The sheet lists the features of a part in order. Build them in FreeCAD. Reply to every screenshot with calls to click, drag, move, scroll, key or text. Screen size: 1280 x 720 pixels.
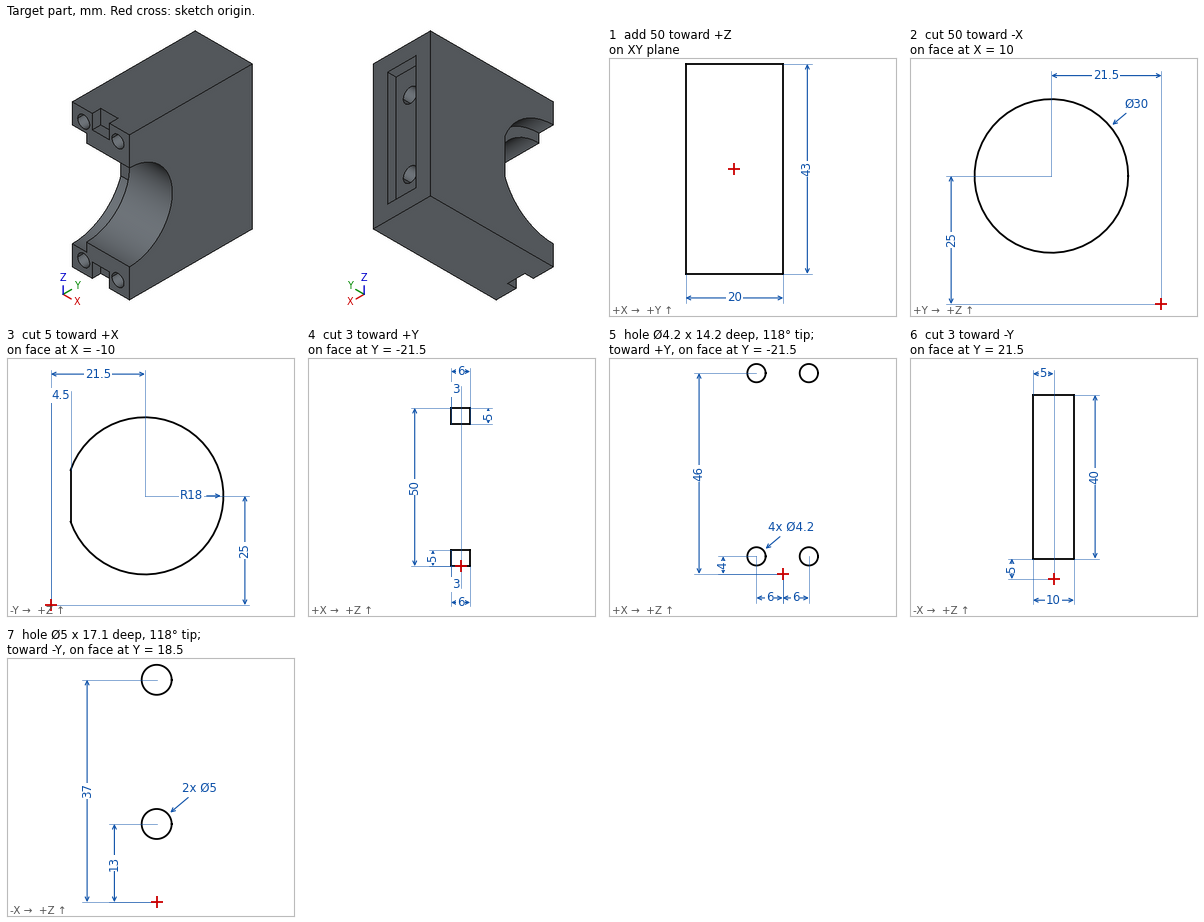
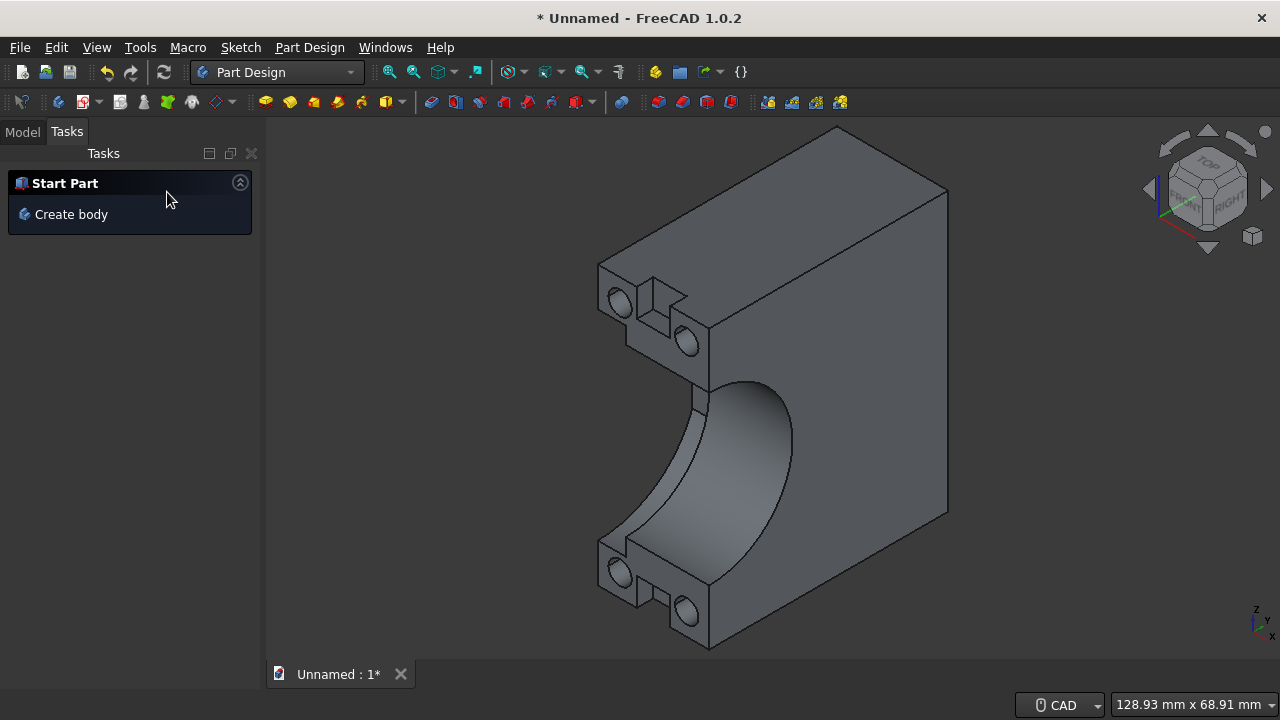
key(4)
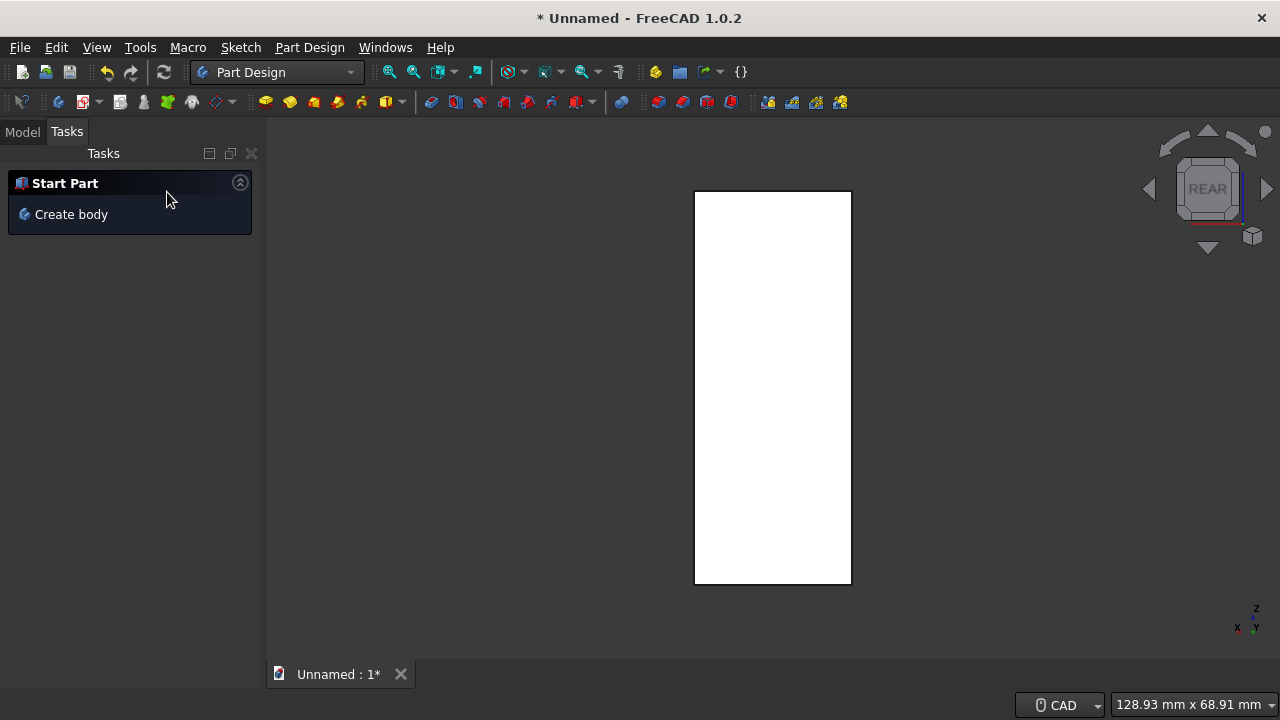
click(773, 275)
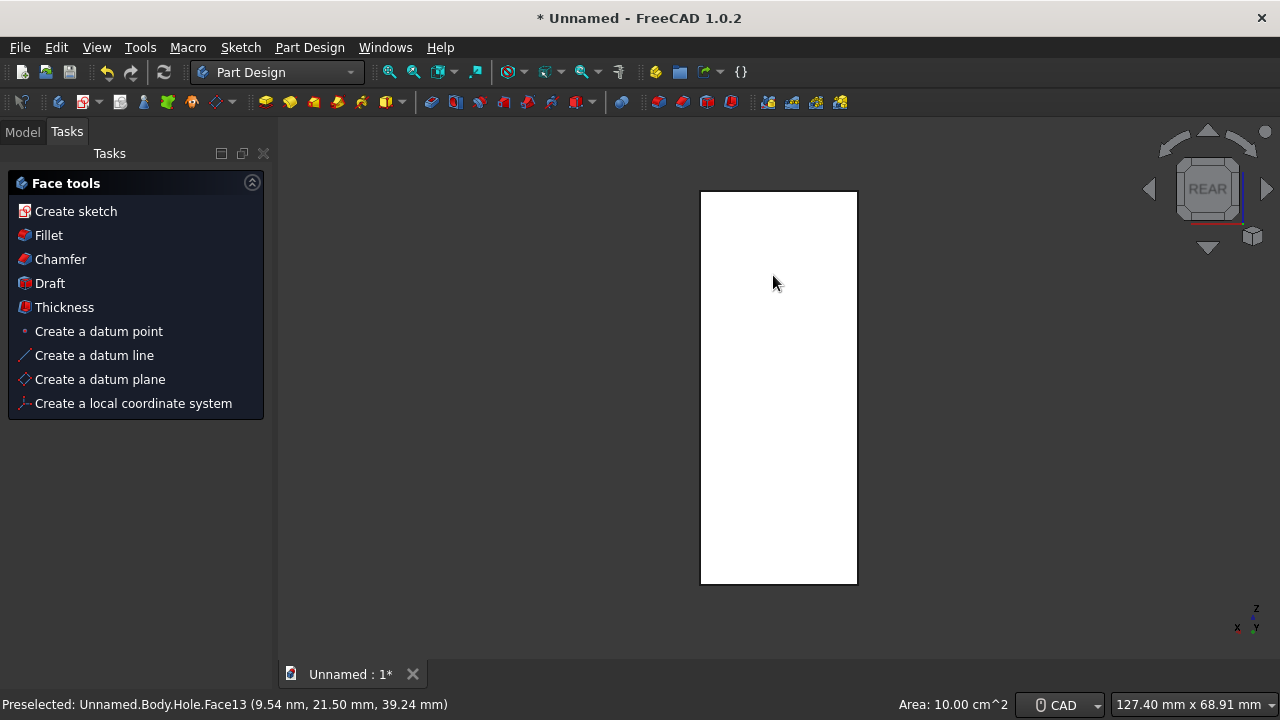
click(84, 102)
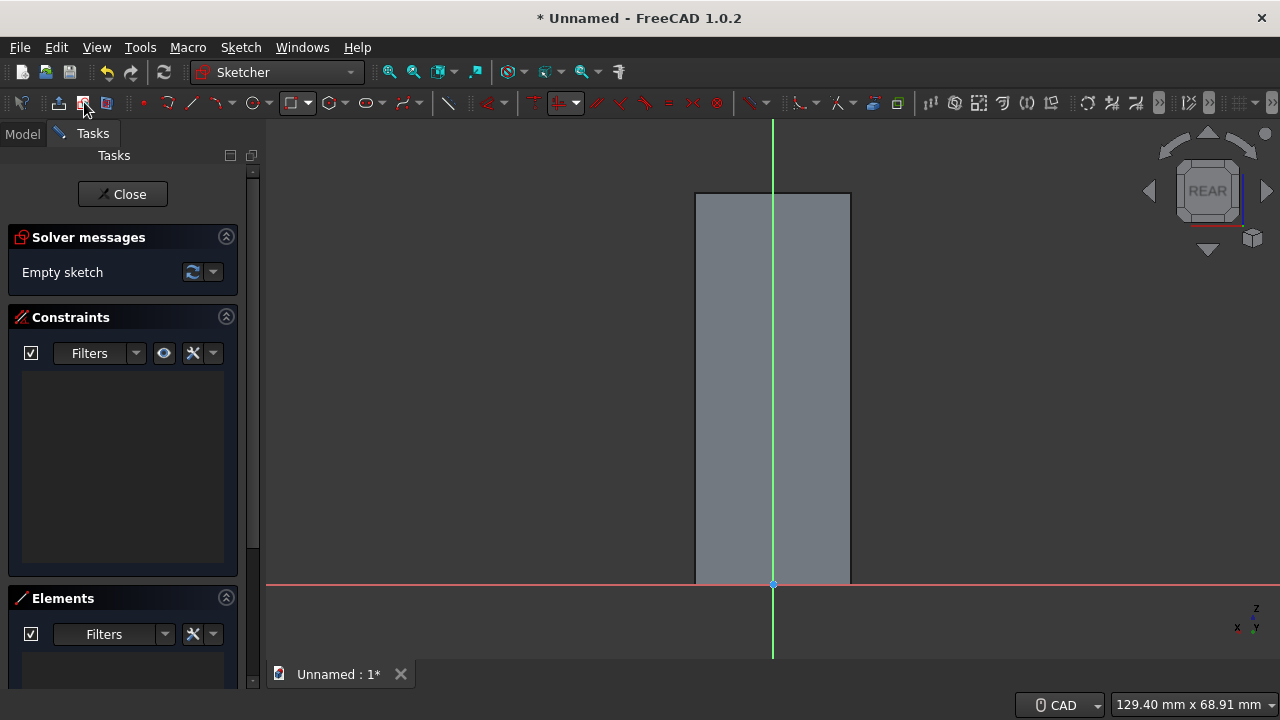
key(g)
key(r)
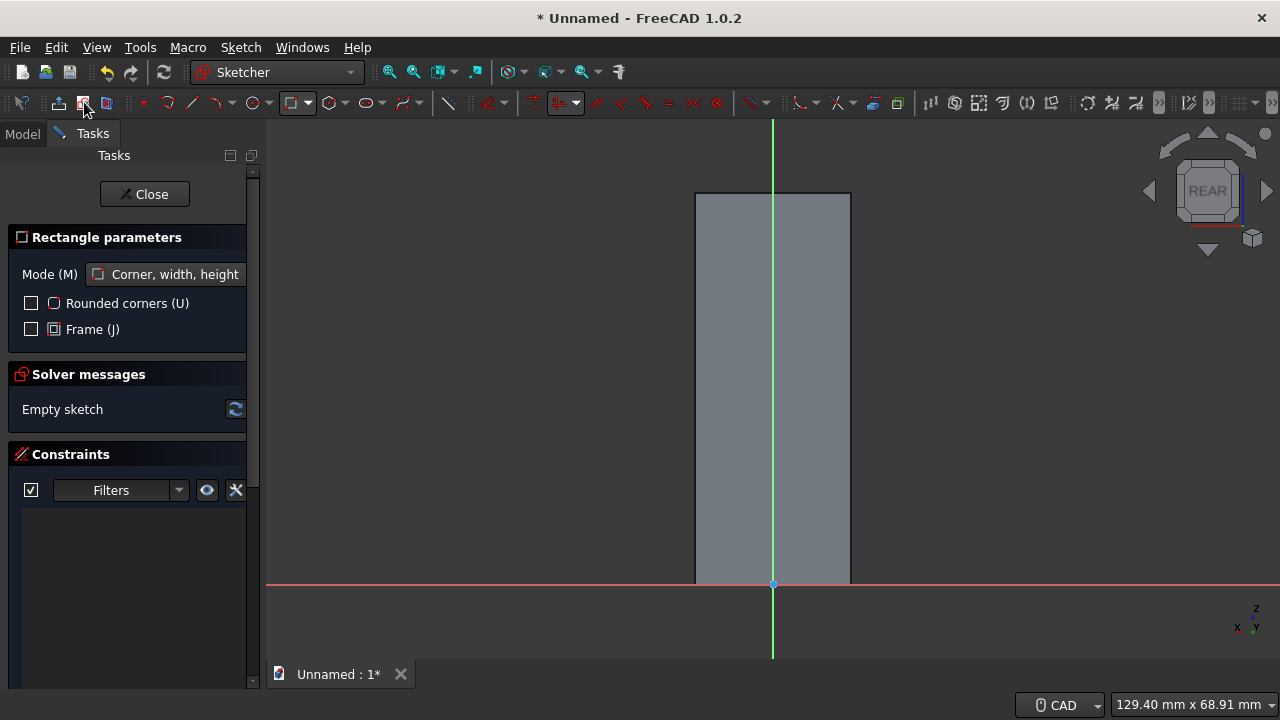
click(734, 232)
move(812, 546)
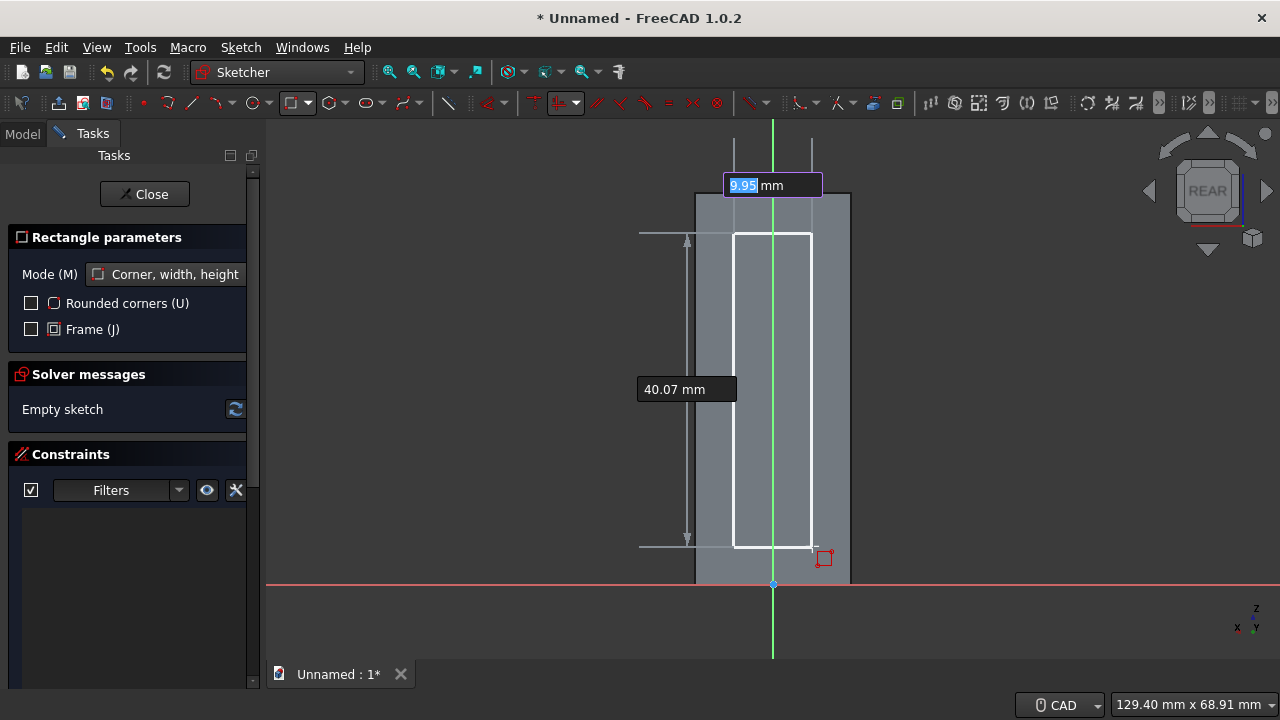
text(10)
key(Tab)
text(40)
key(Return)
key(Escape)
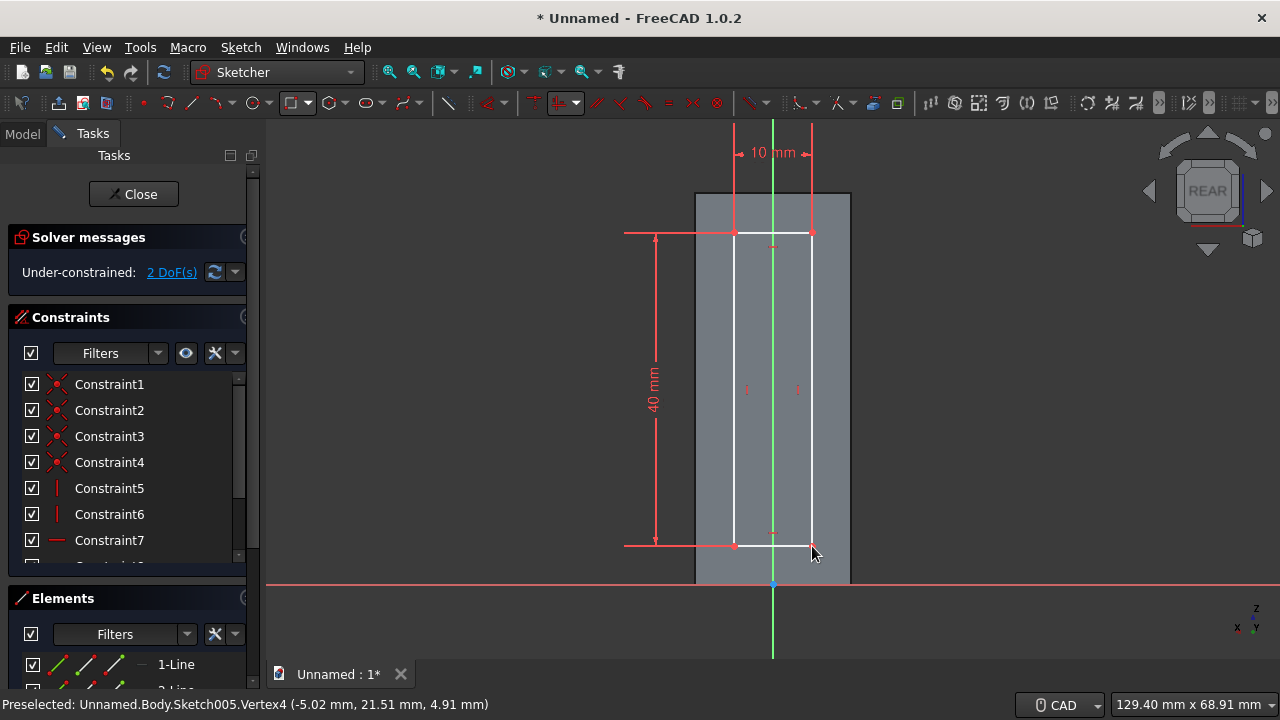
click(488, 104)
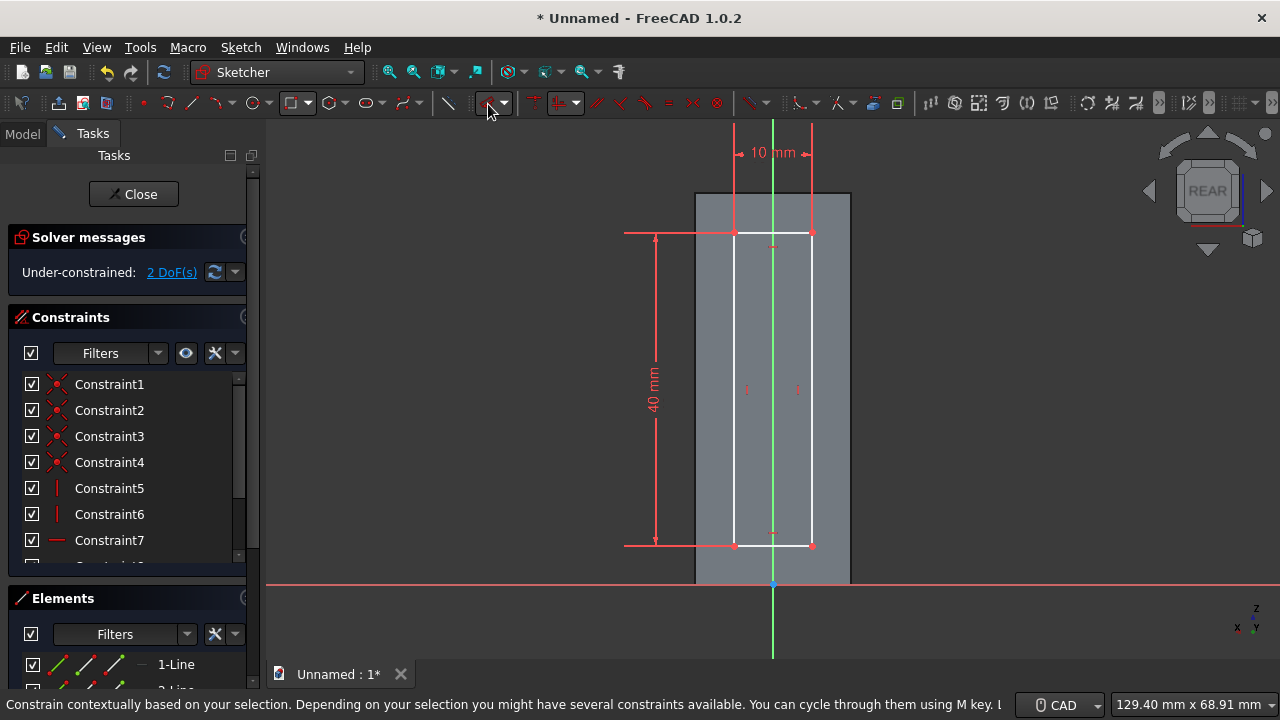
click(734, 233)
click(754, 619)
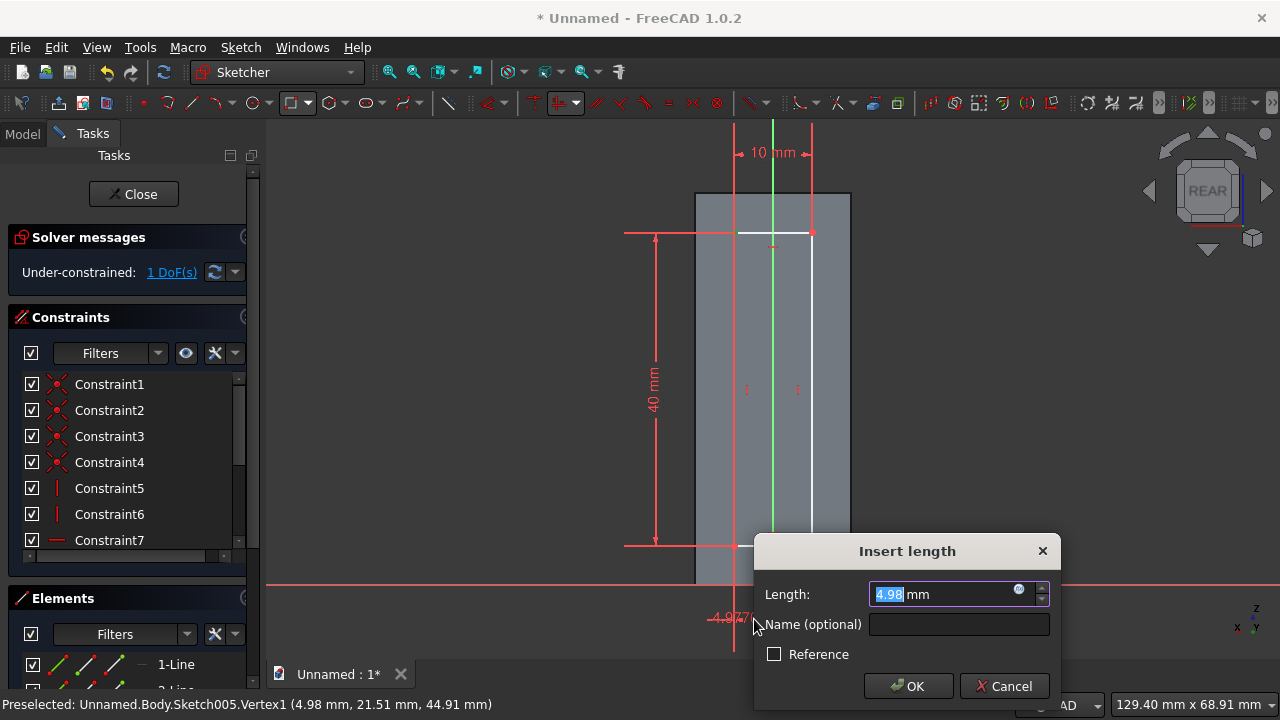
text(5)
key(Return)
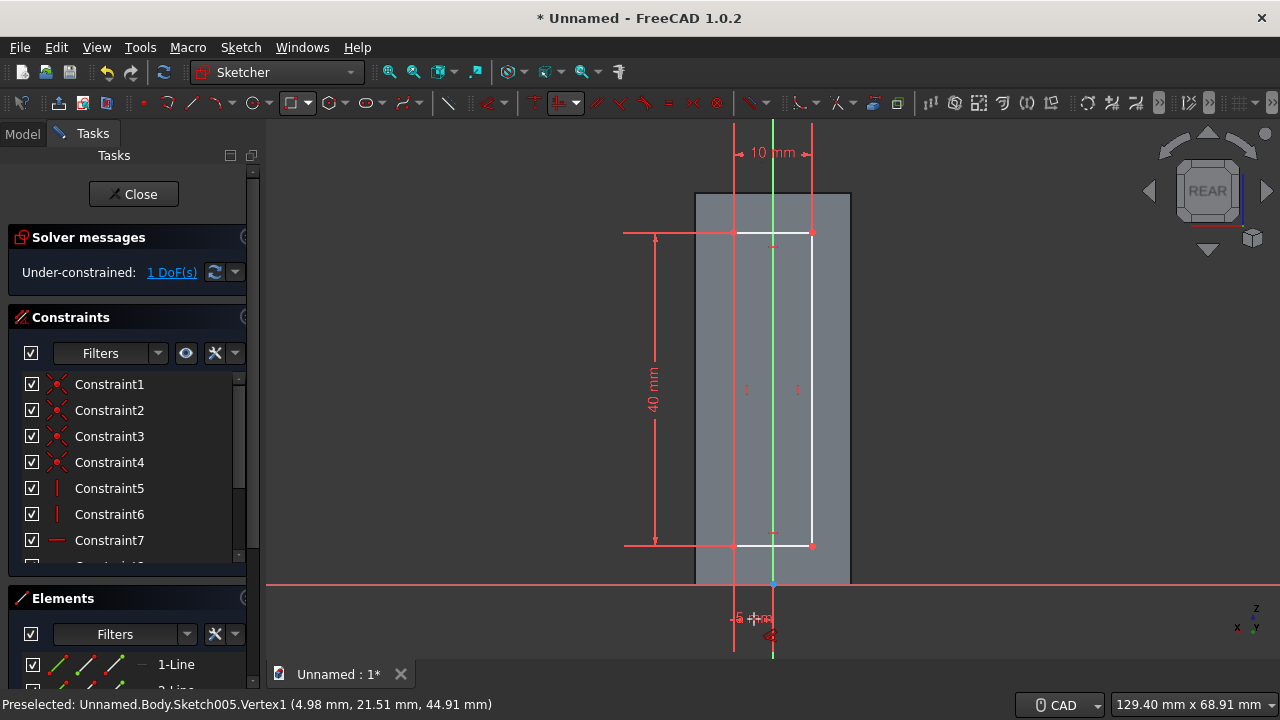
click(734, 546)
click(700, 566)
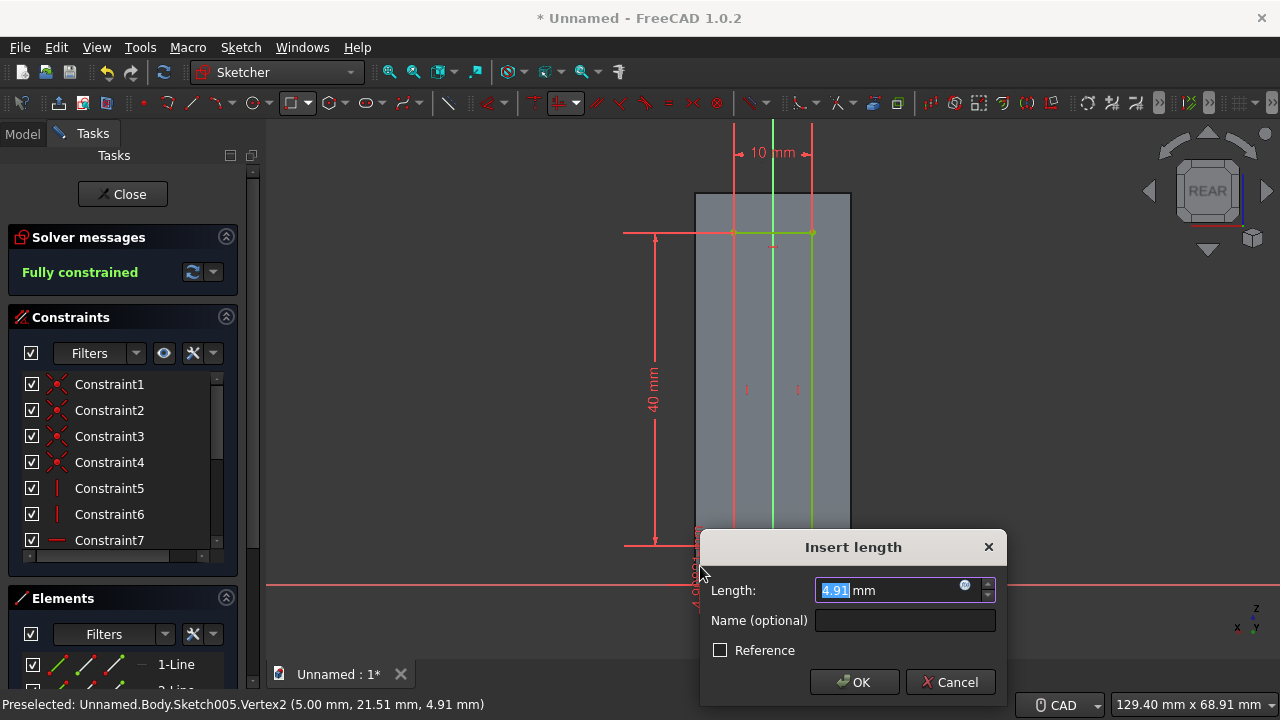
text(5)
key(Return)
key(Escape)